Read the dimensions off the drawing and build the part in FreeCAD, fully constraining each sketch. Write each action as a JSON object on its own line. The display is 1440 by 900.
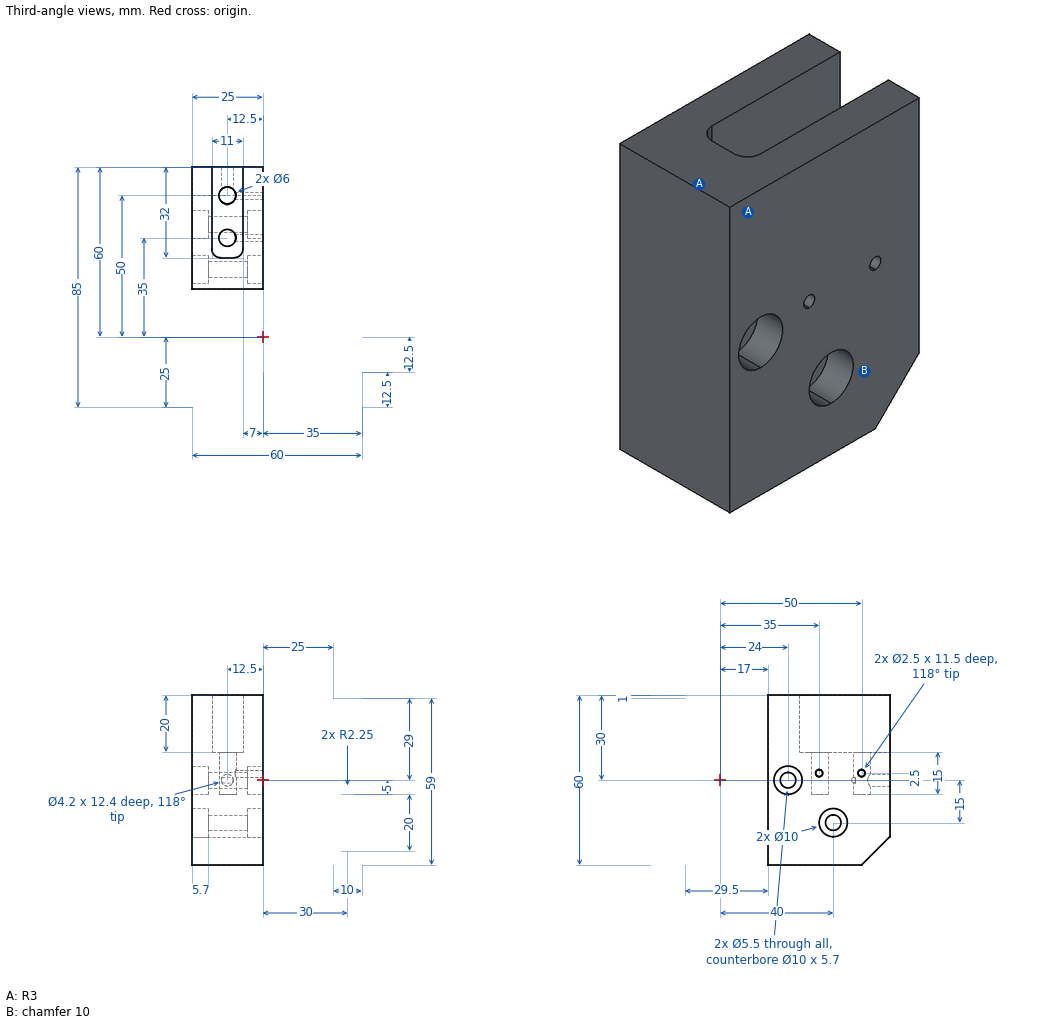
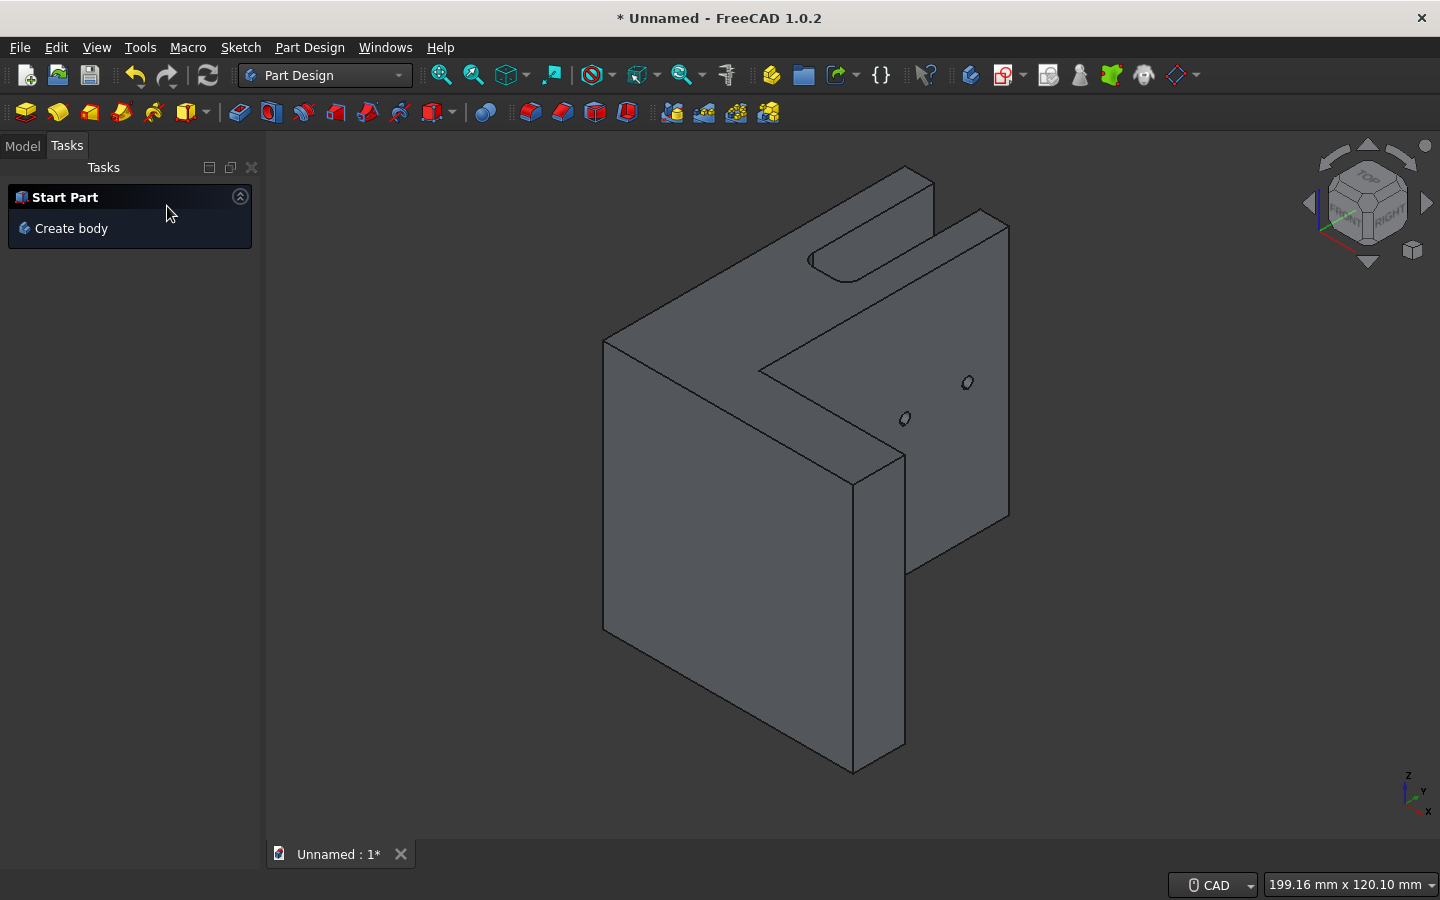
{"action": "key", "text": "4"}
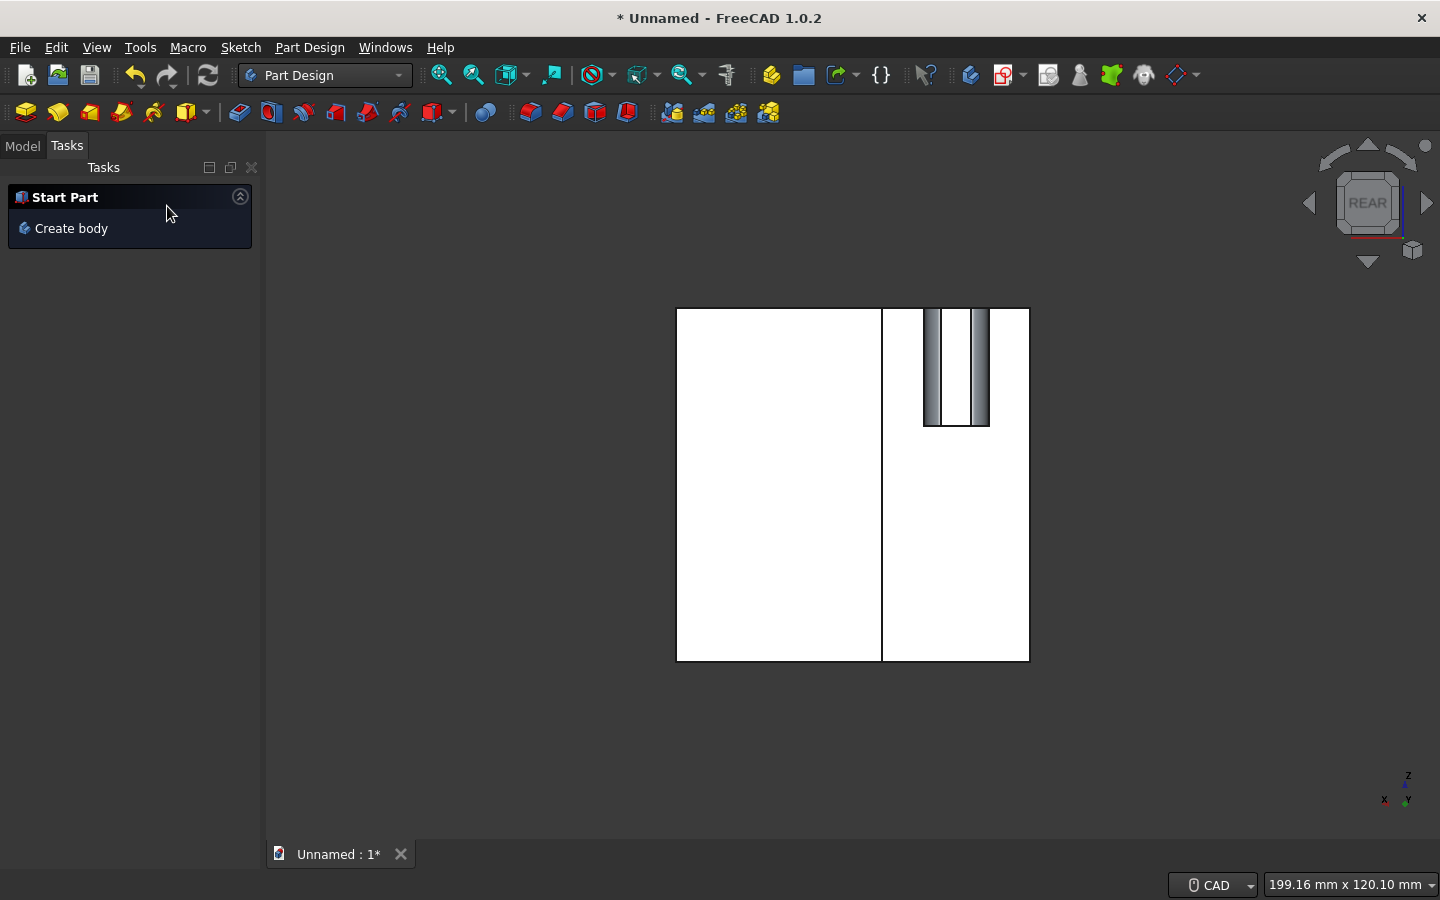
{"action": "left_click", "coordinate": [956, 535]}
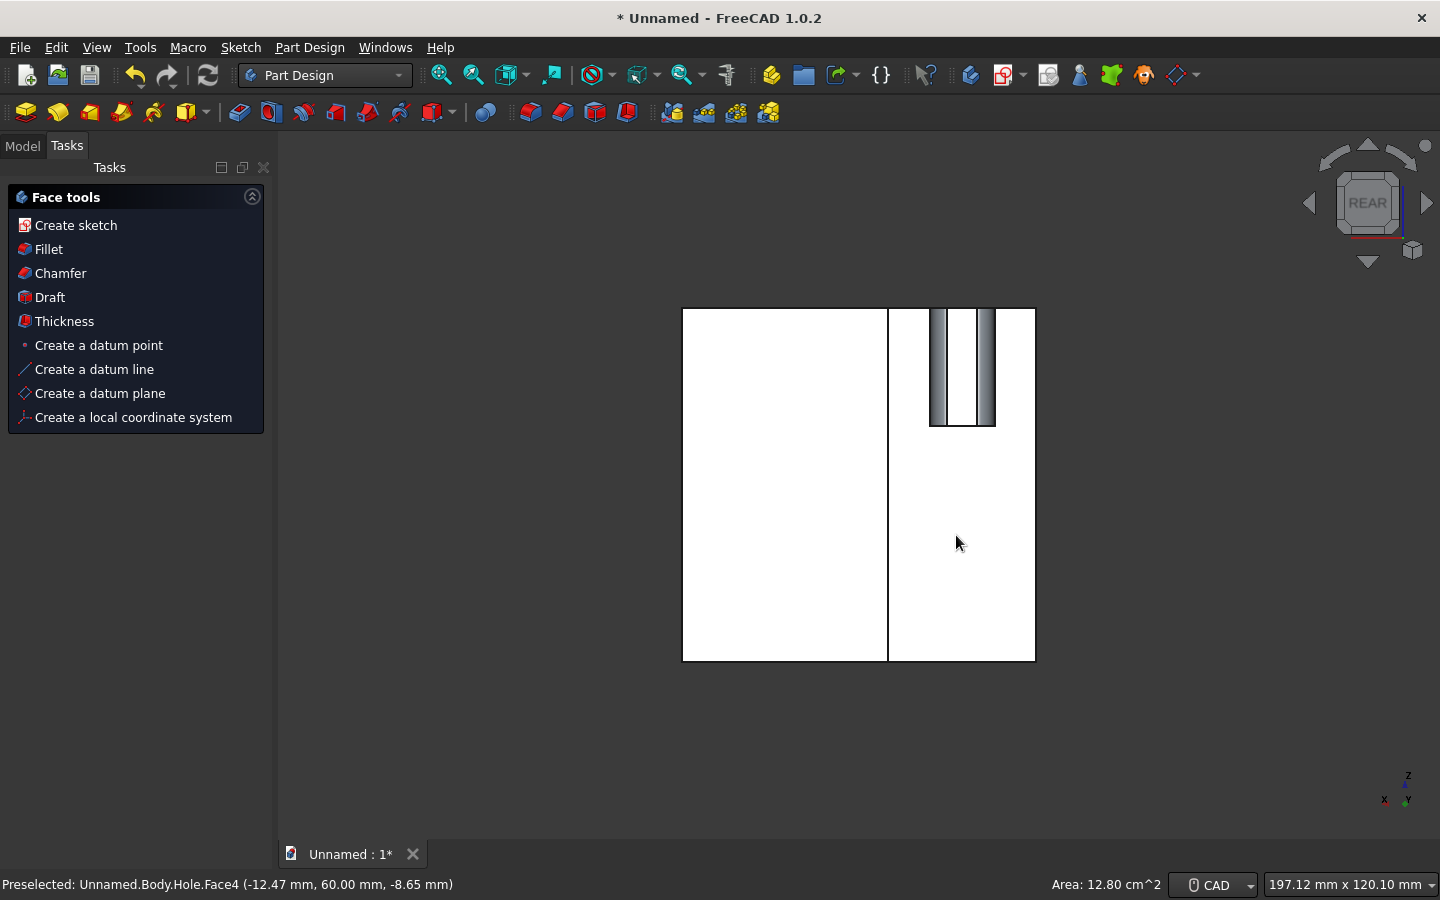
{"action": "left_click", "coordinate": [1004, 76]}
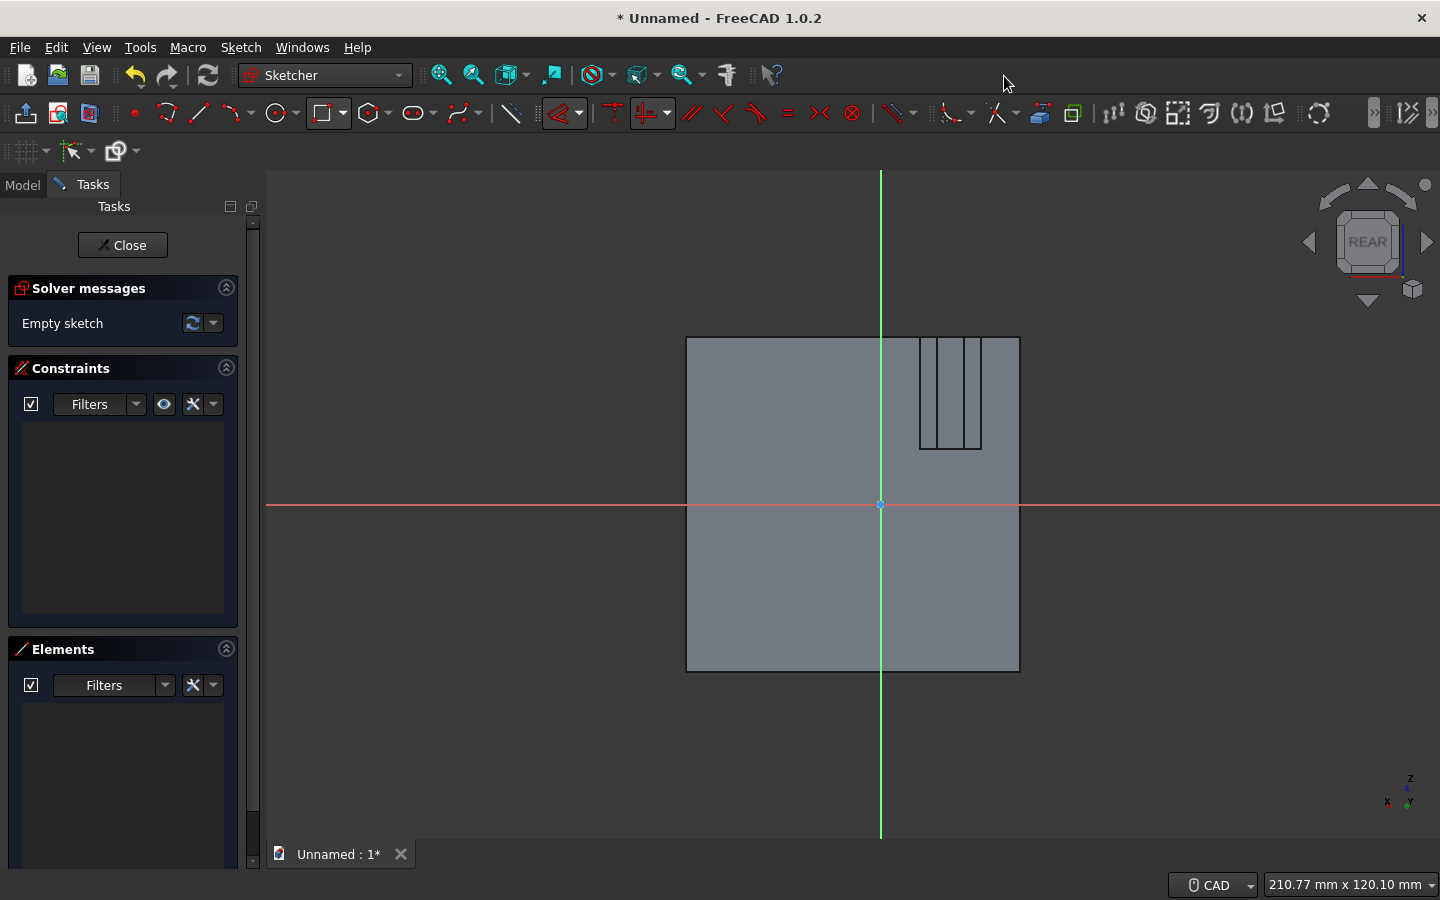
{"action": "scroll", "coordinate": [959, 505], "scroll_direction": "up", "scroll_amount": 15}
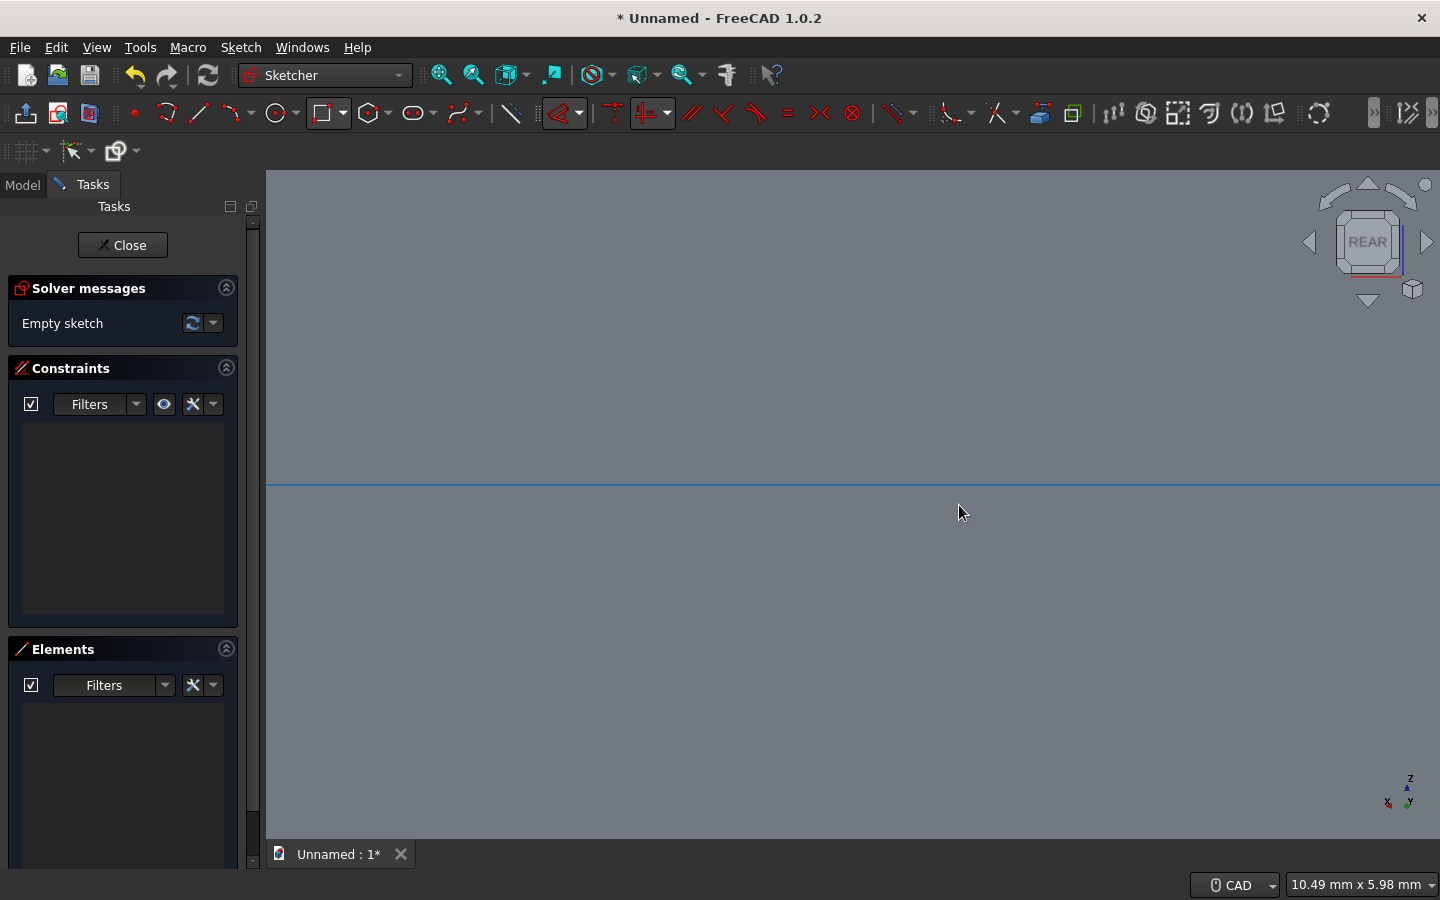
{"action": "left_click", "coordinate": [276, 114]}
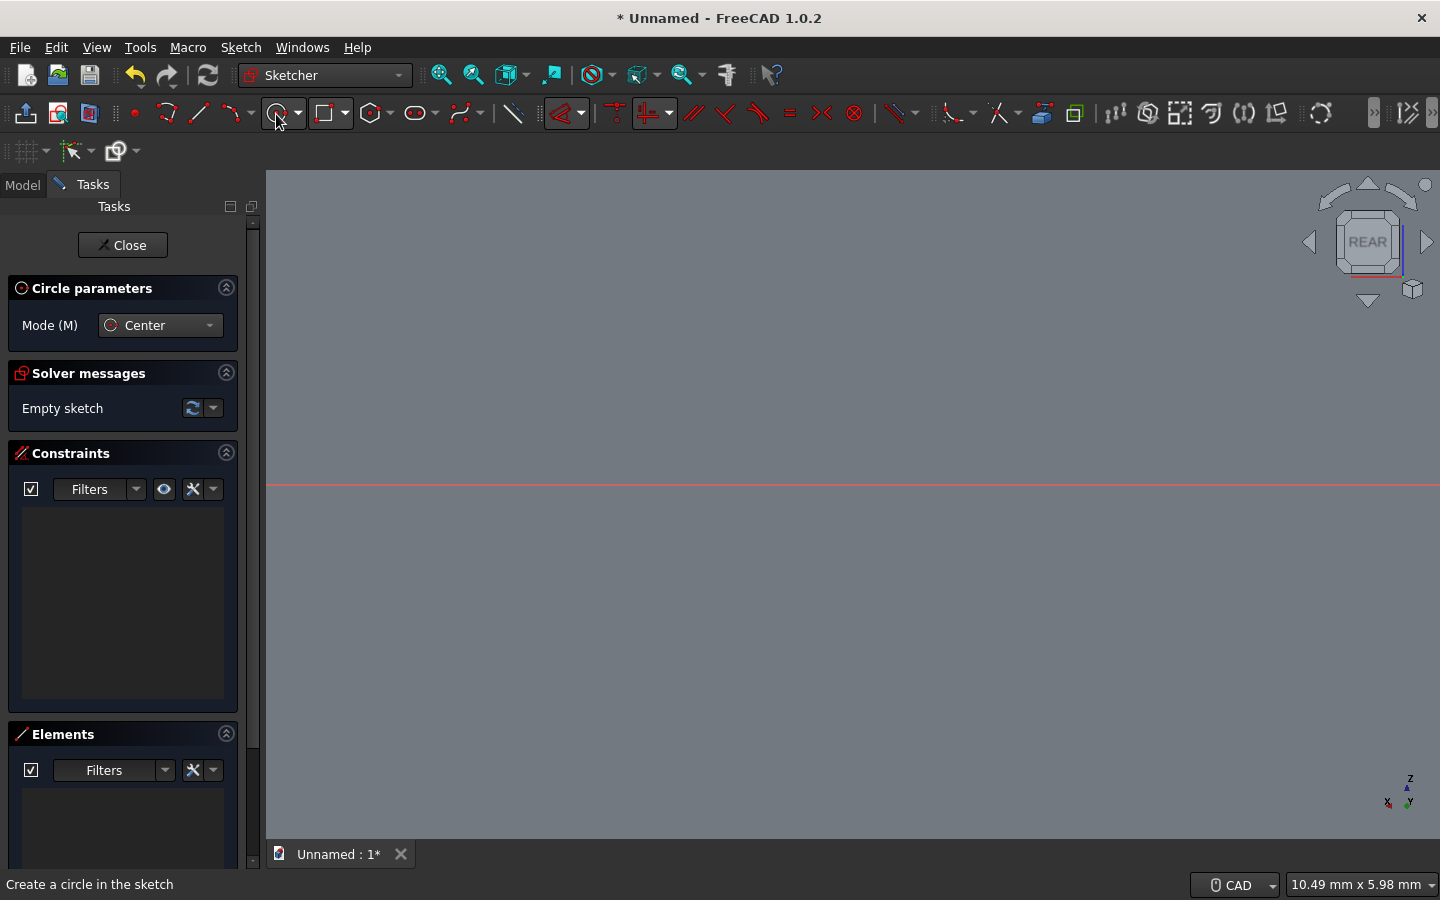
{"action": "left_click", "coordinate": [777, 485]}
{"action": "mouse_move", "coordinate": [943, 319]}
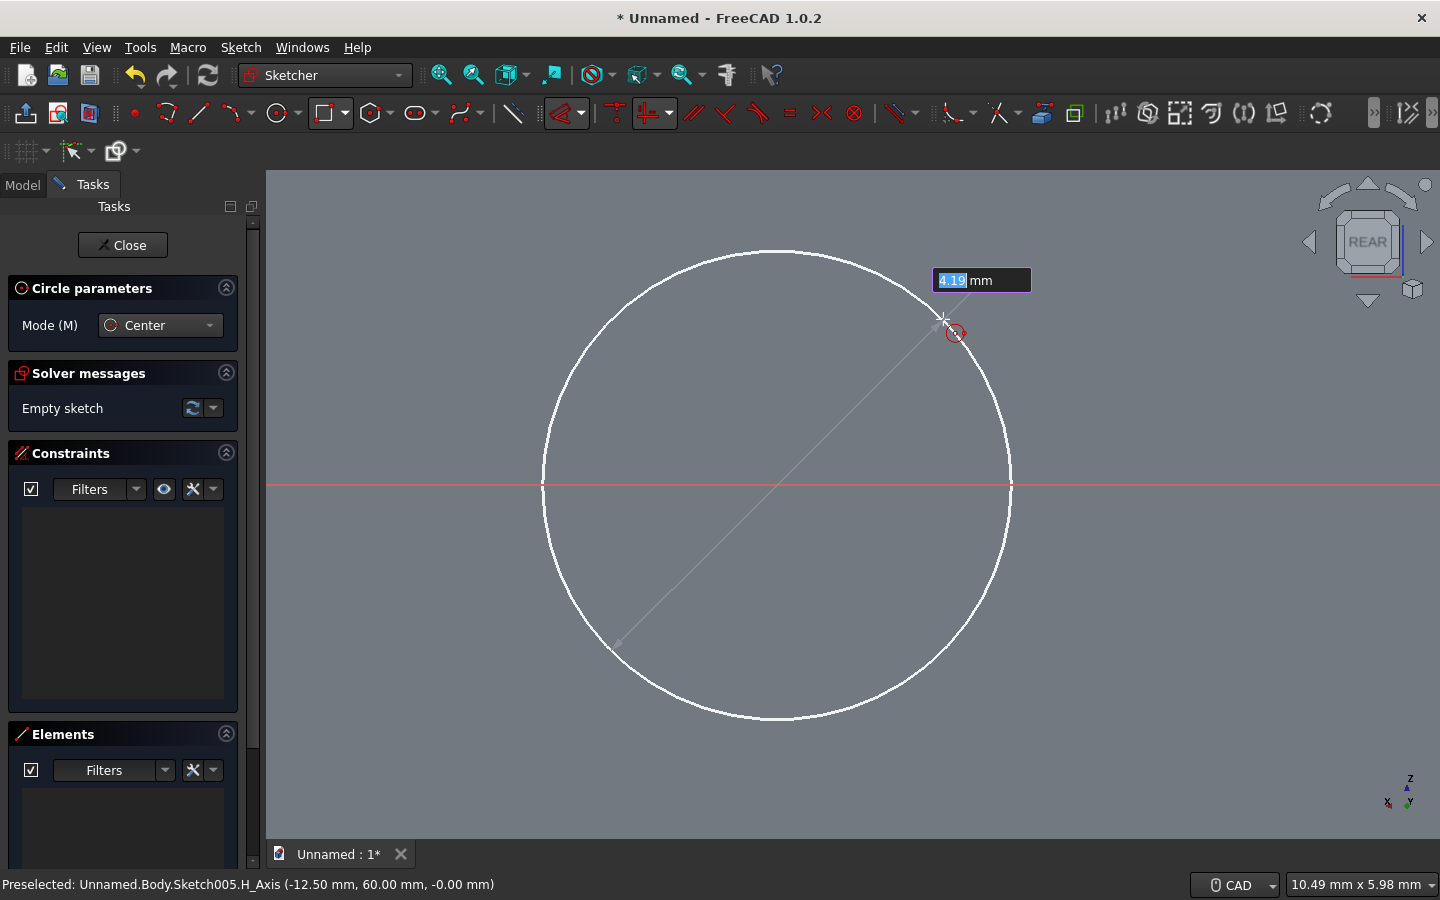
{"action": "type", "text": "4.2"}
{"action": "key", "text": "Return"}
{"action": "key", "text": "Escape"}